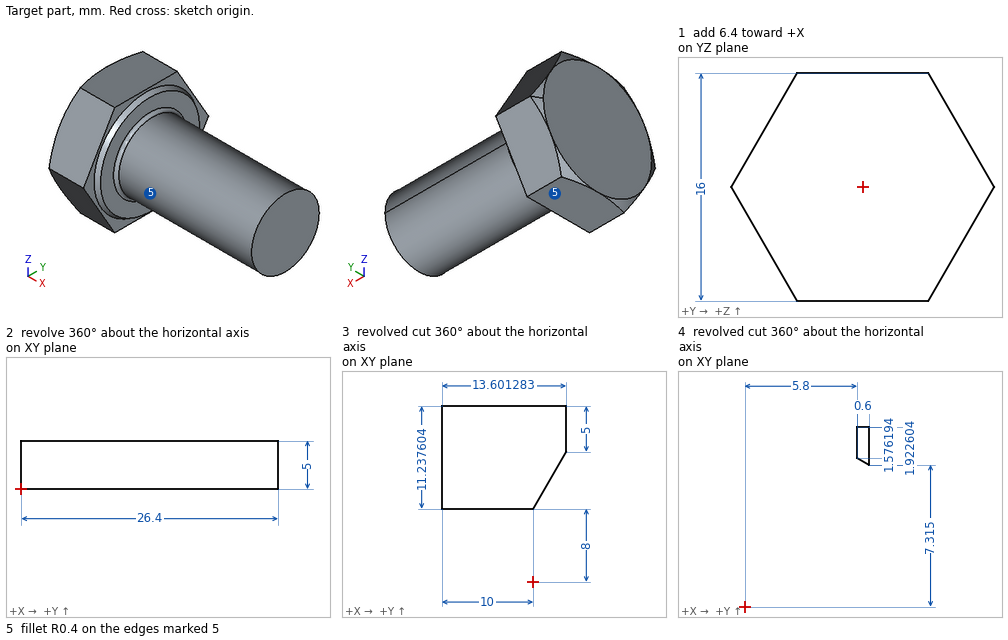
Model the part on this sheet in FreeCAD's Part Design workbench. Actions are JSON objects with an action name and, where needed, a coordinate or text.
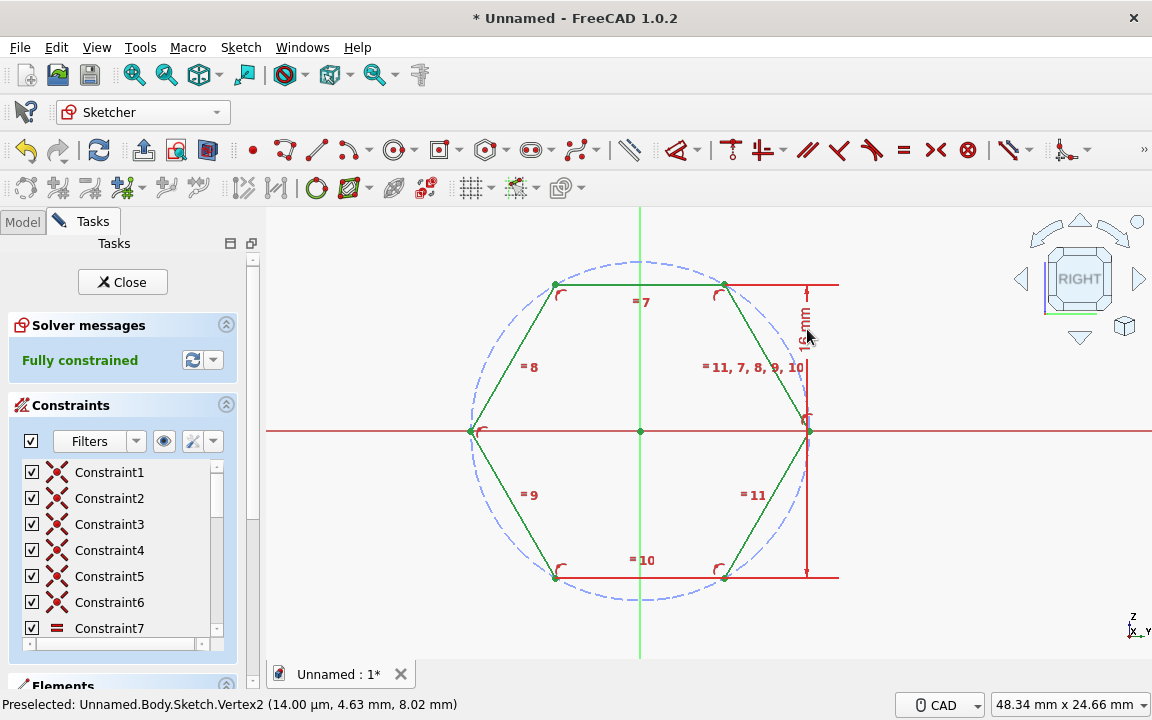
{"action": "left_click", "coordinate": [123, 282]}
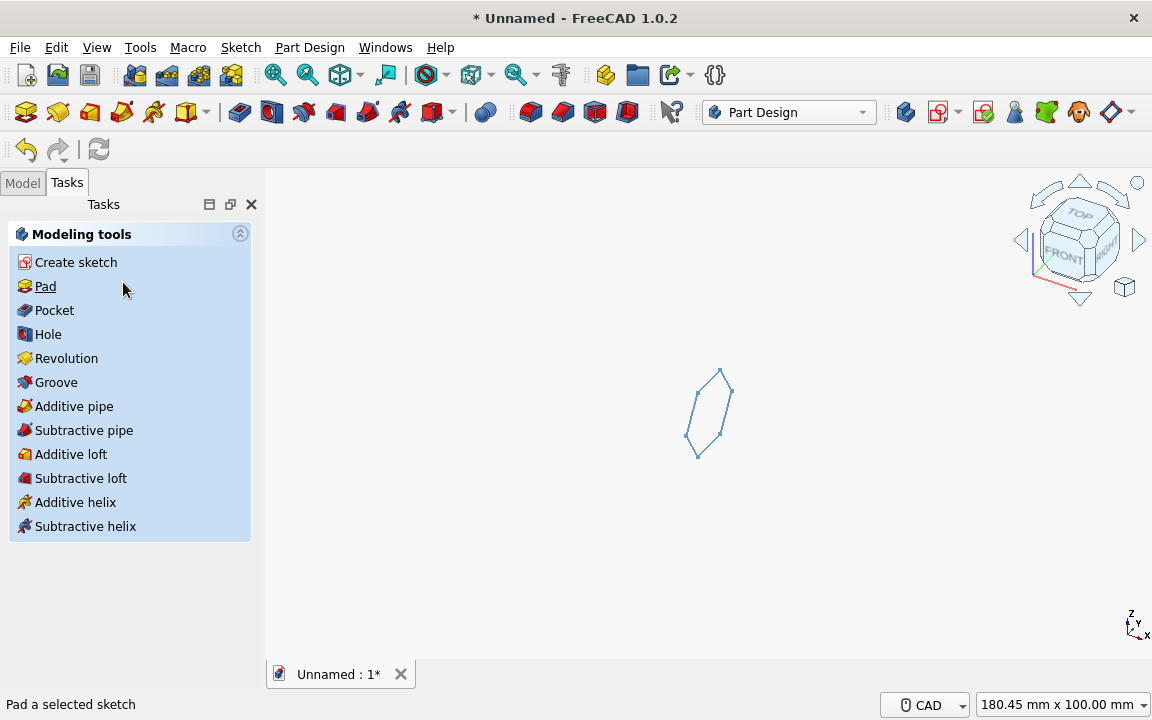
{"action": "left_click", "coordinate": [26, 112]}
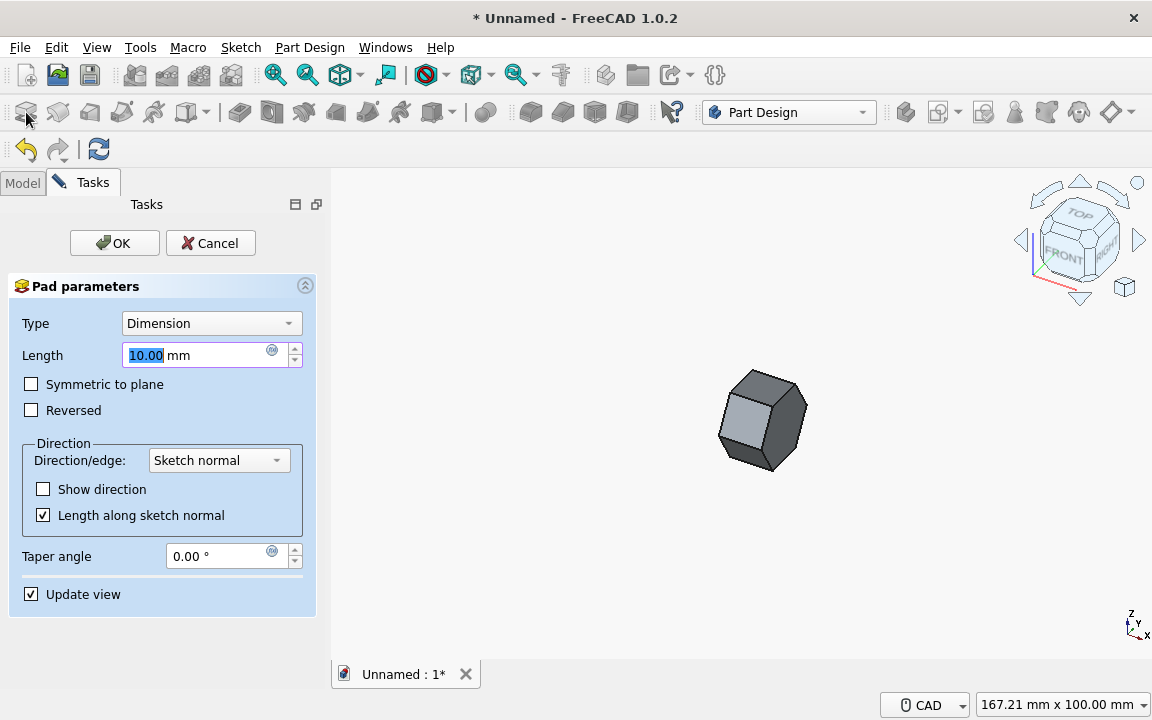
{"action": "type", "text": "6.4"}
{"action": "key", "text": "Tab"}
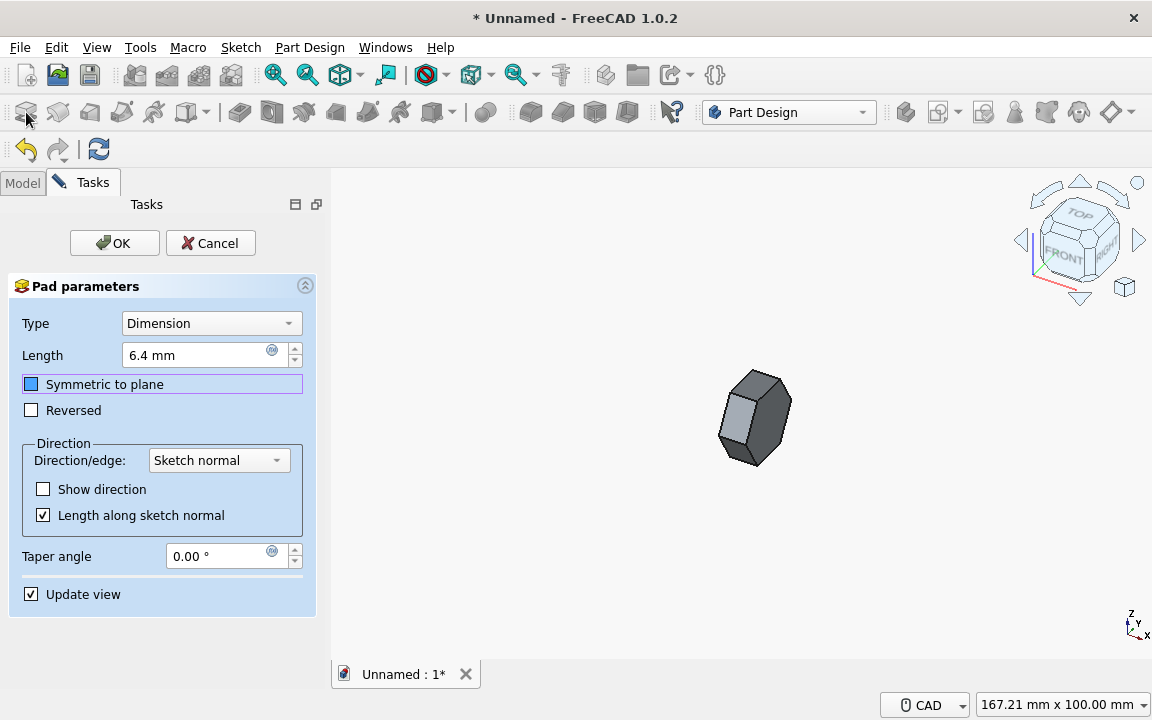
{"action": "left_click", "coordinate": [115, 243]}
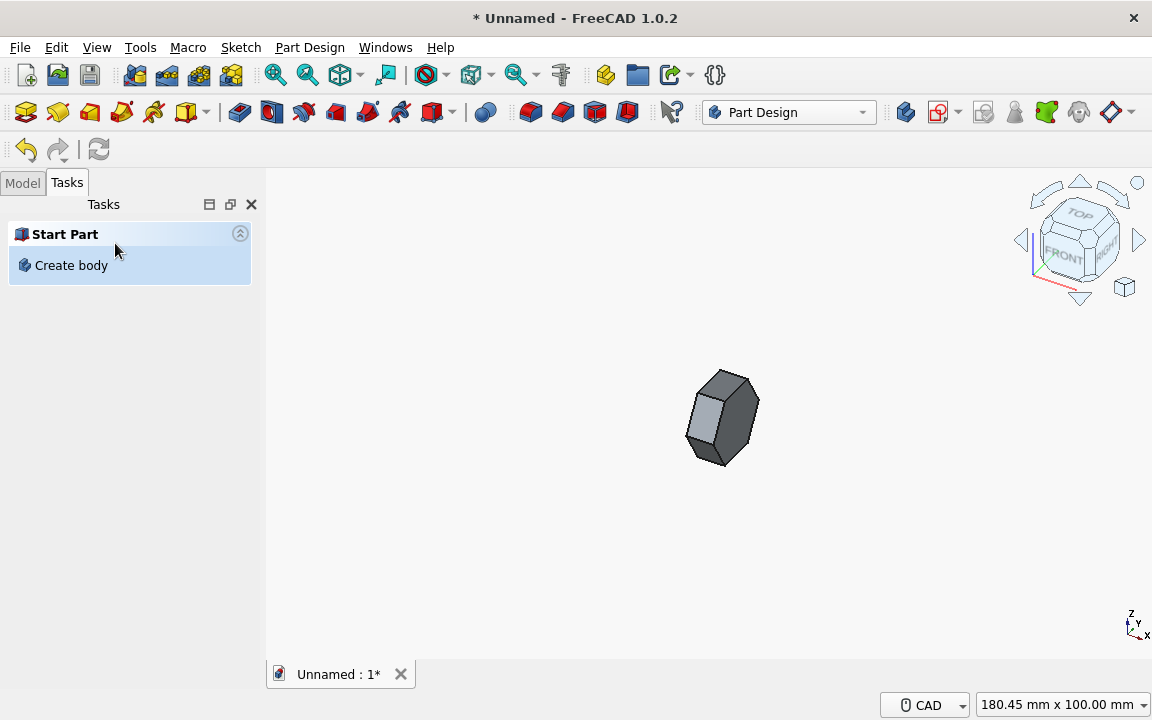
{"action": "left_click", "coordinate": [276, 76]}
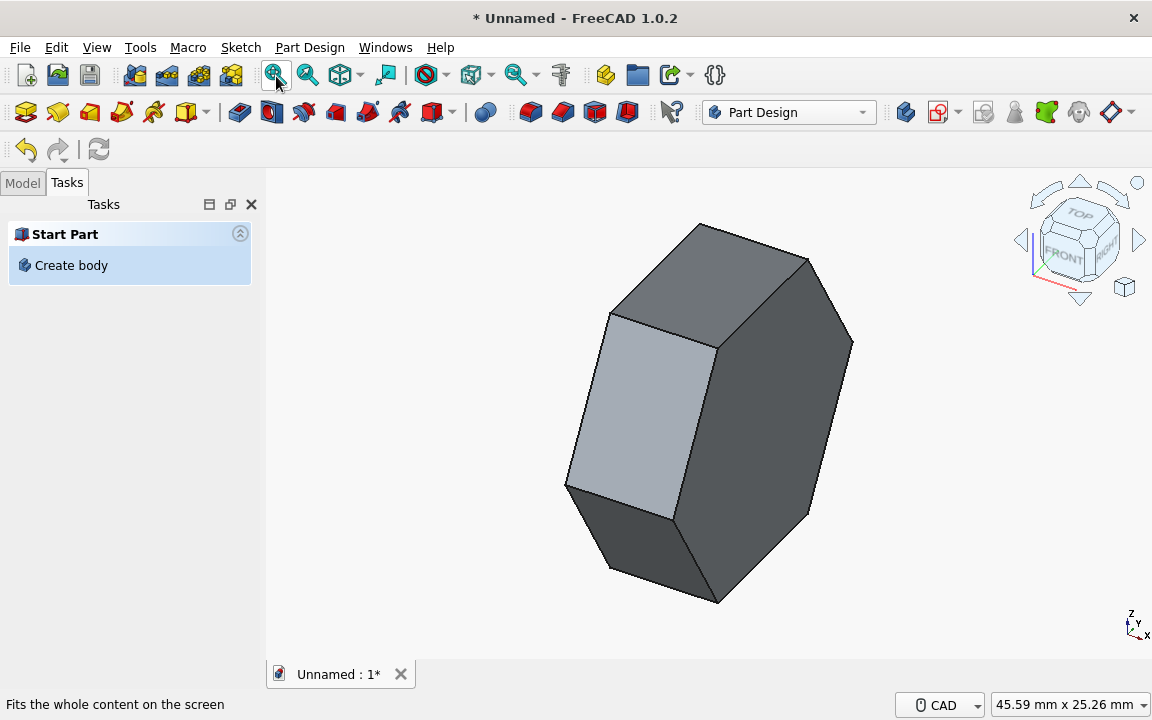
{"action": "left_click", "coordinate": [938, 112]}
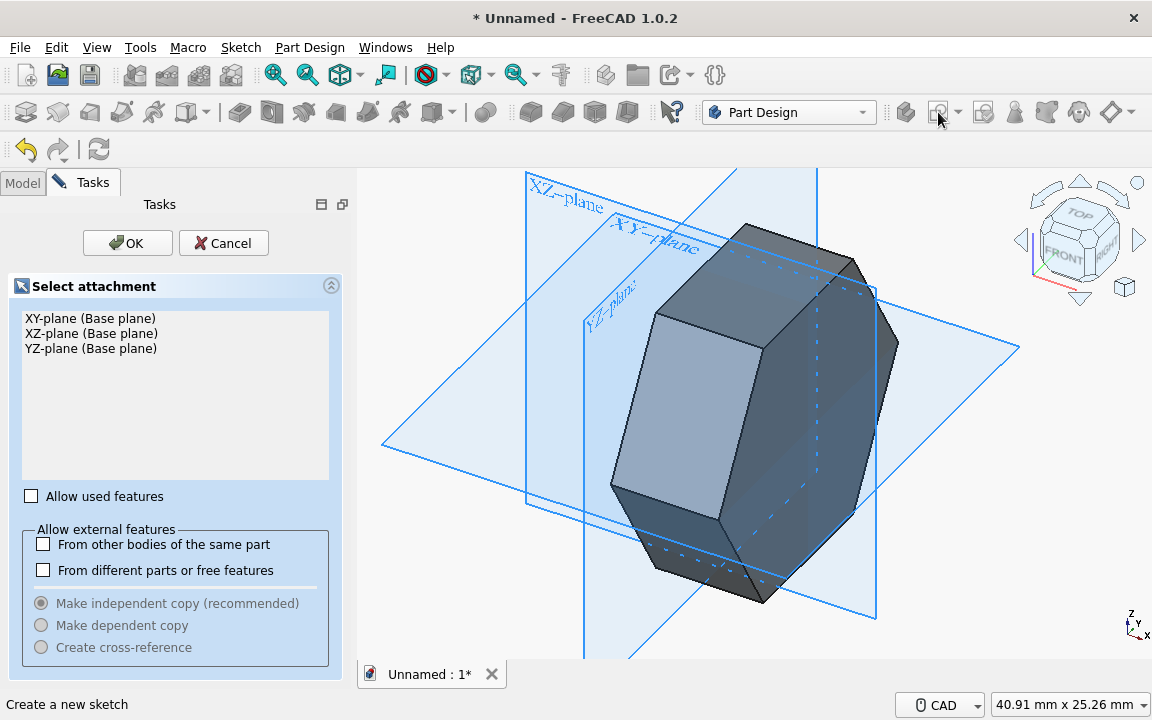
{"action": "left_click", "coordinate": [82, 318]}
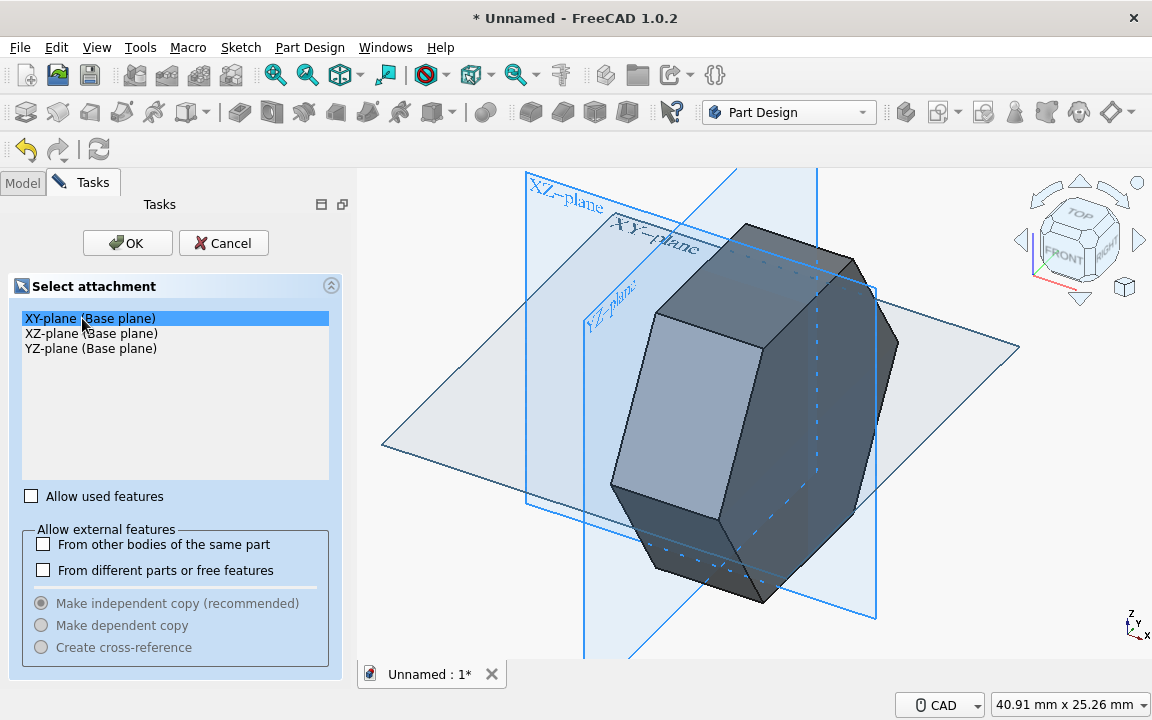
{"action": "left_click", "coordinate": [128, 243]}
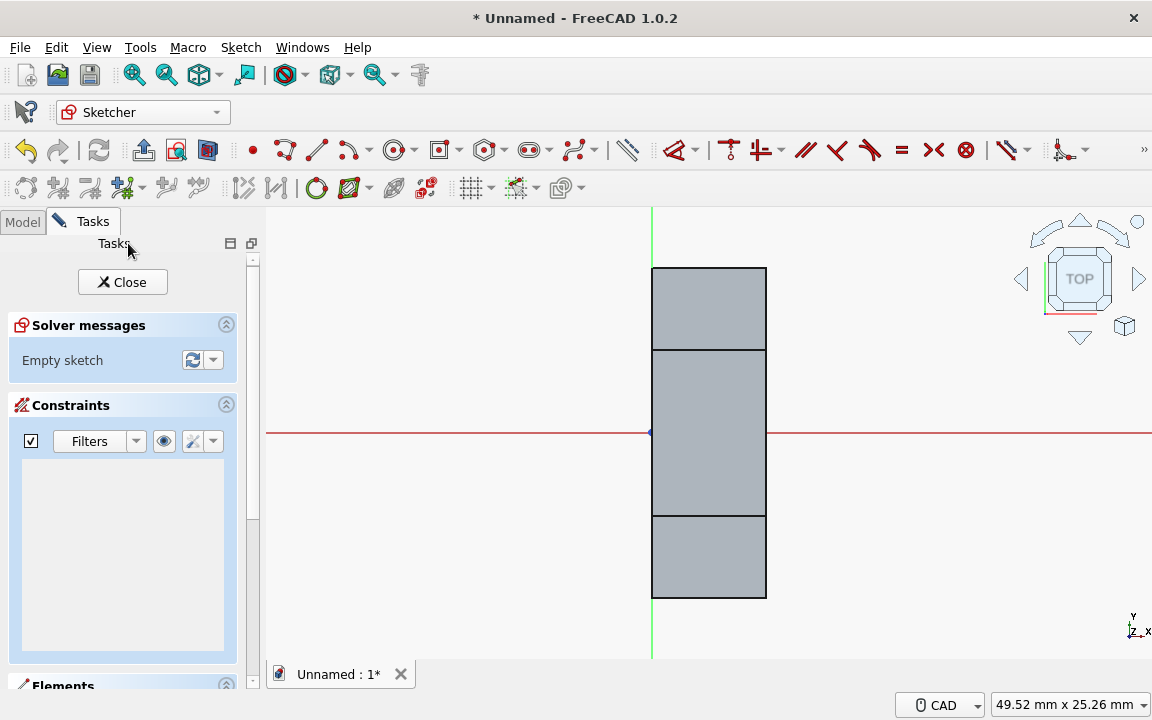
{"action": "left_click", "coordinate": [208, 150]}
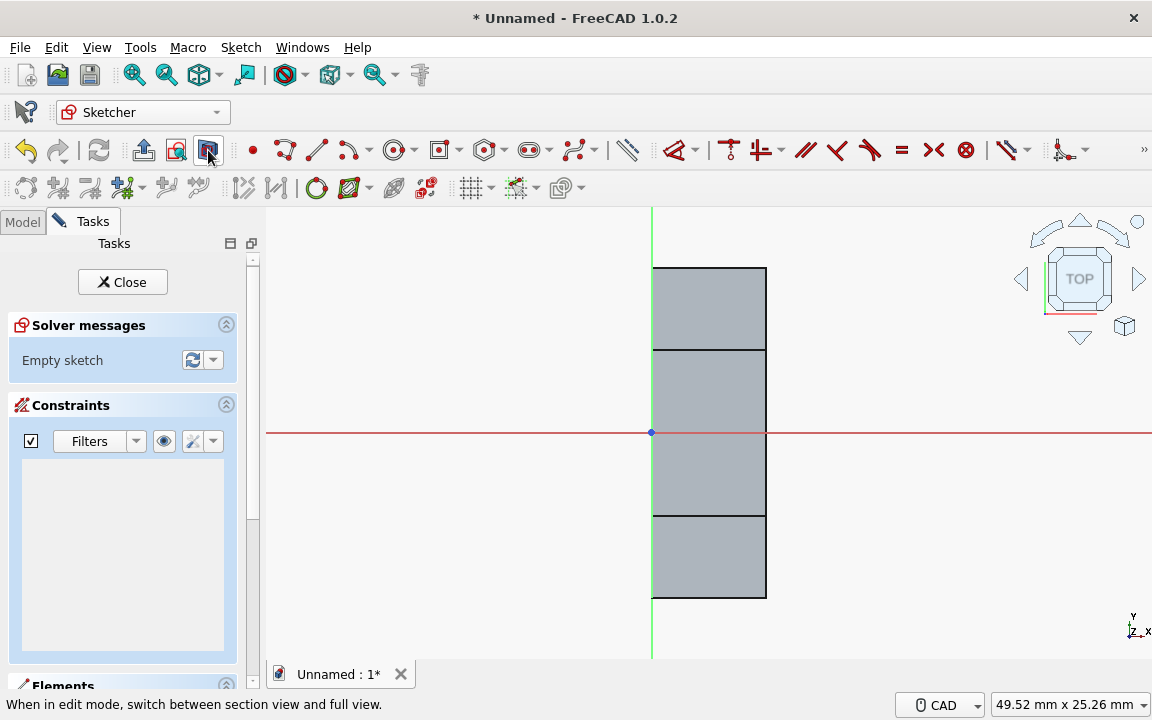
{"action": "scroll", "coordinate": [294, 524], "scroll_direction": "down", "scroll_amount": 2}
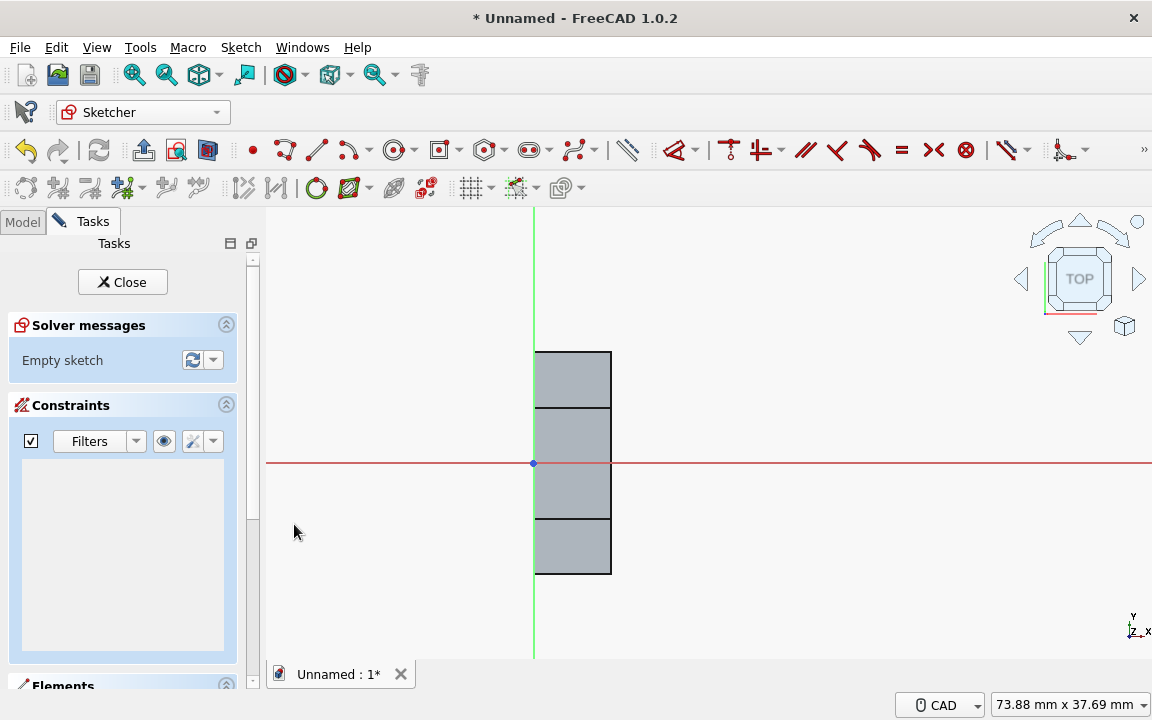
{"action": "scroll", "coordinate": [797, 434], "scroll_direction": "up", "scroll_amount": 2}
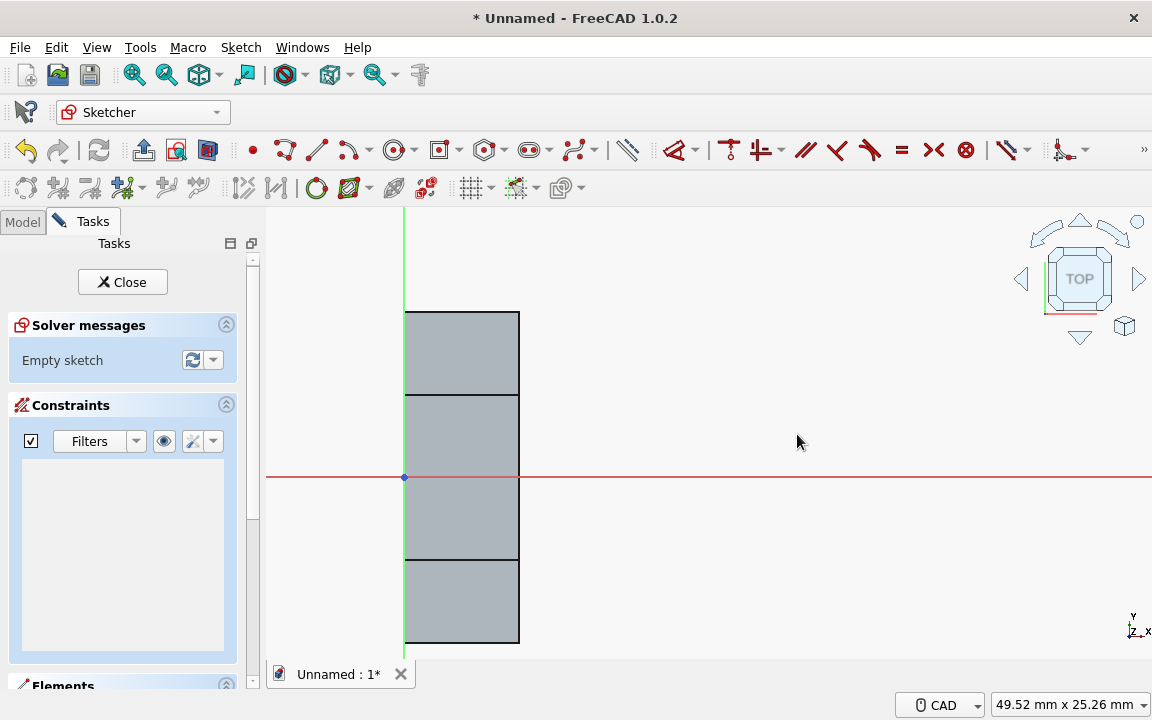
{"action": "key", "text": "g r"}